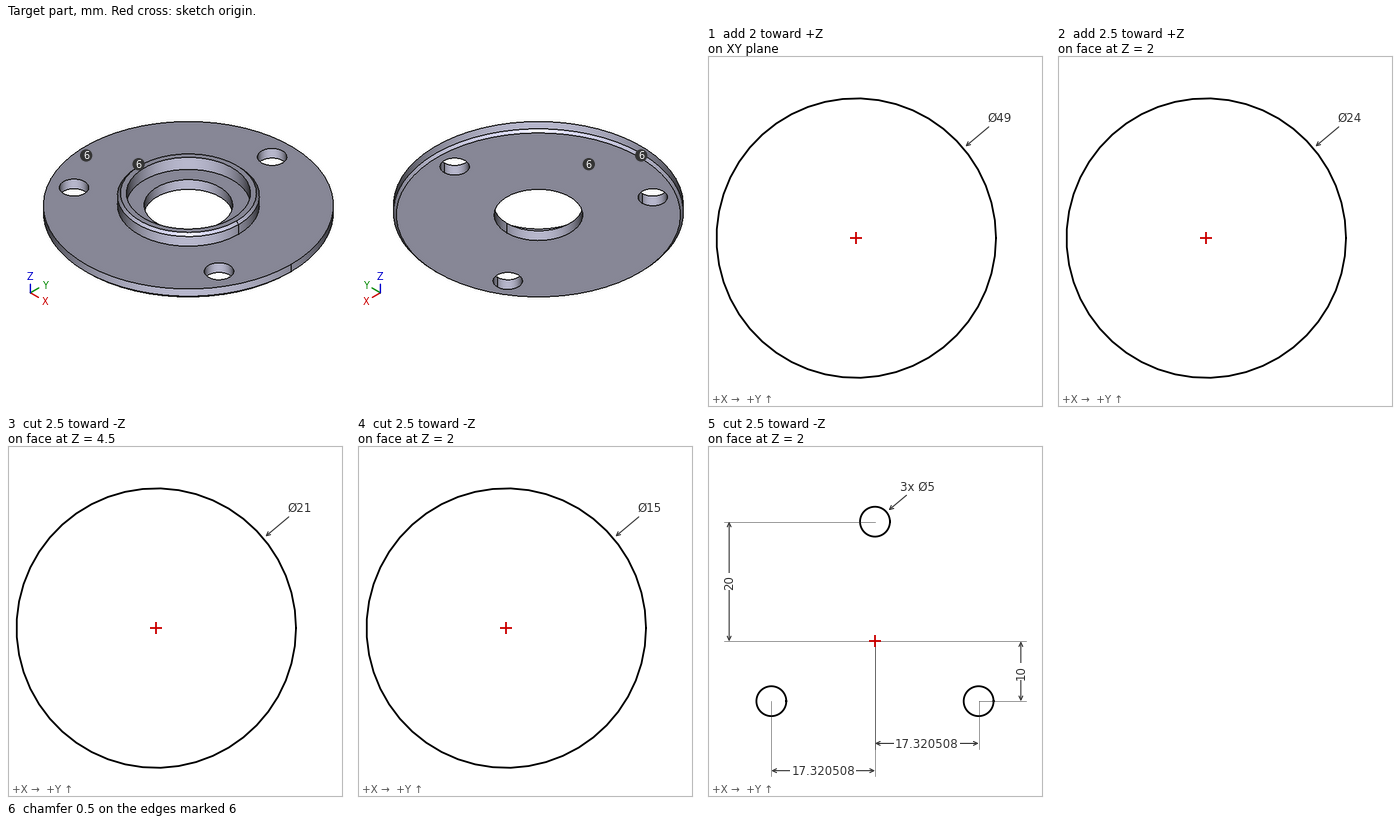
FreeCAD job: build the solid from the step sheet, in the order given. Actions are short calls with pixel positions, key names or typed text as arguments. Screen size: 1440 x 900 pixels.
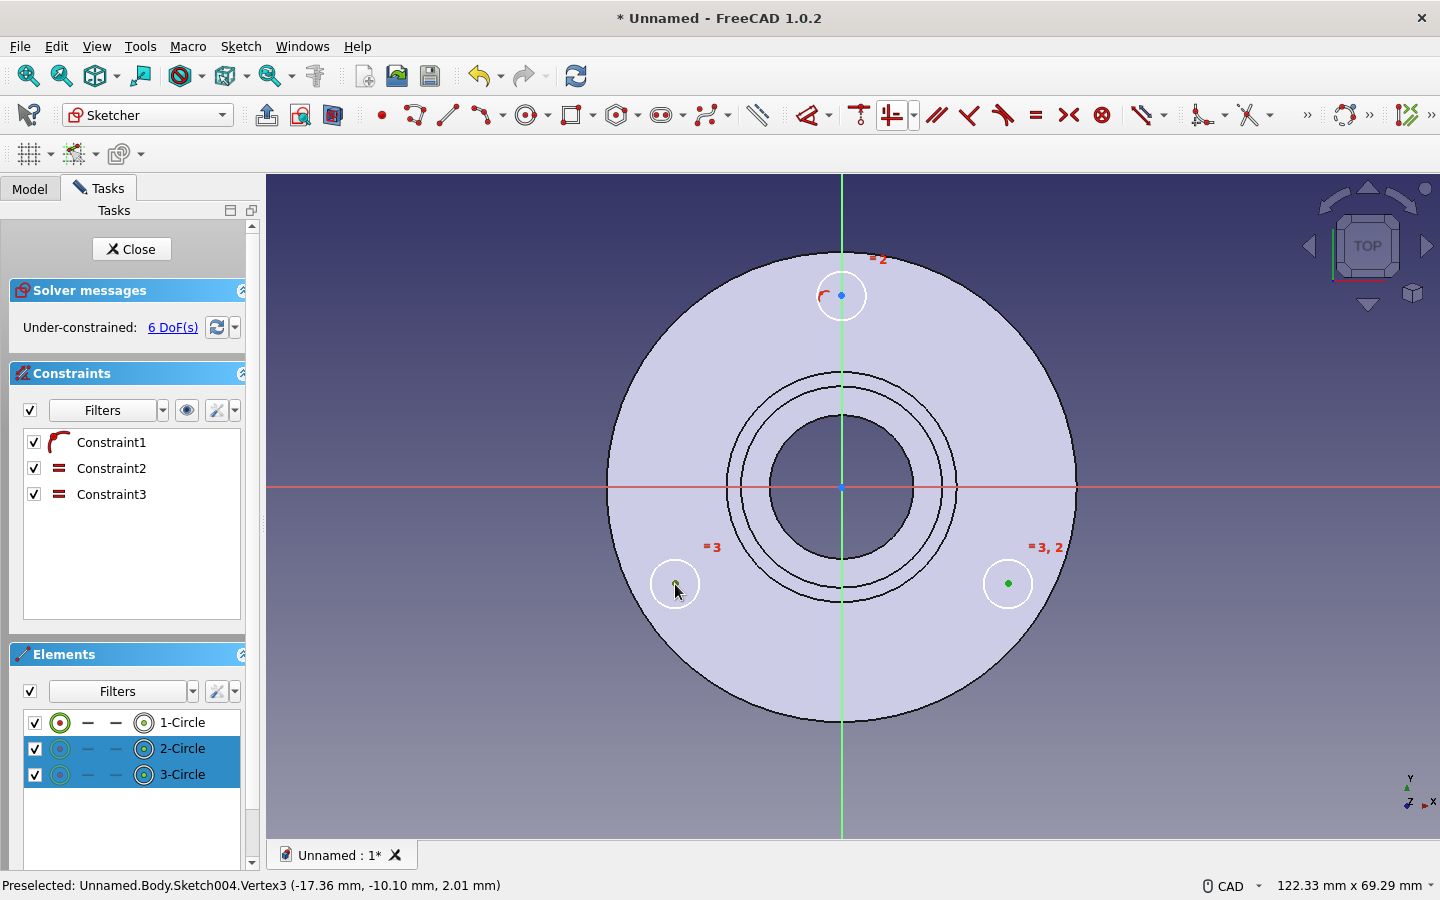
key(h)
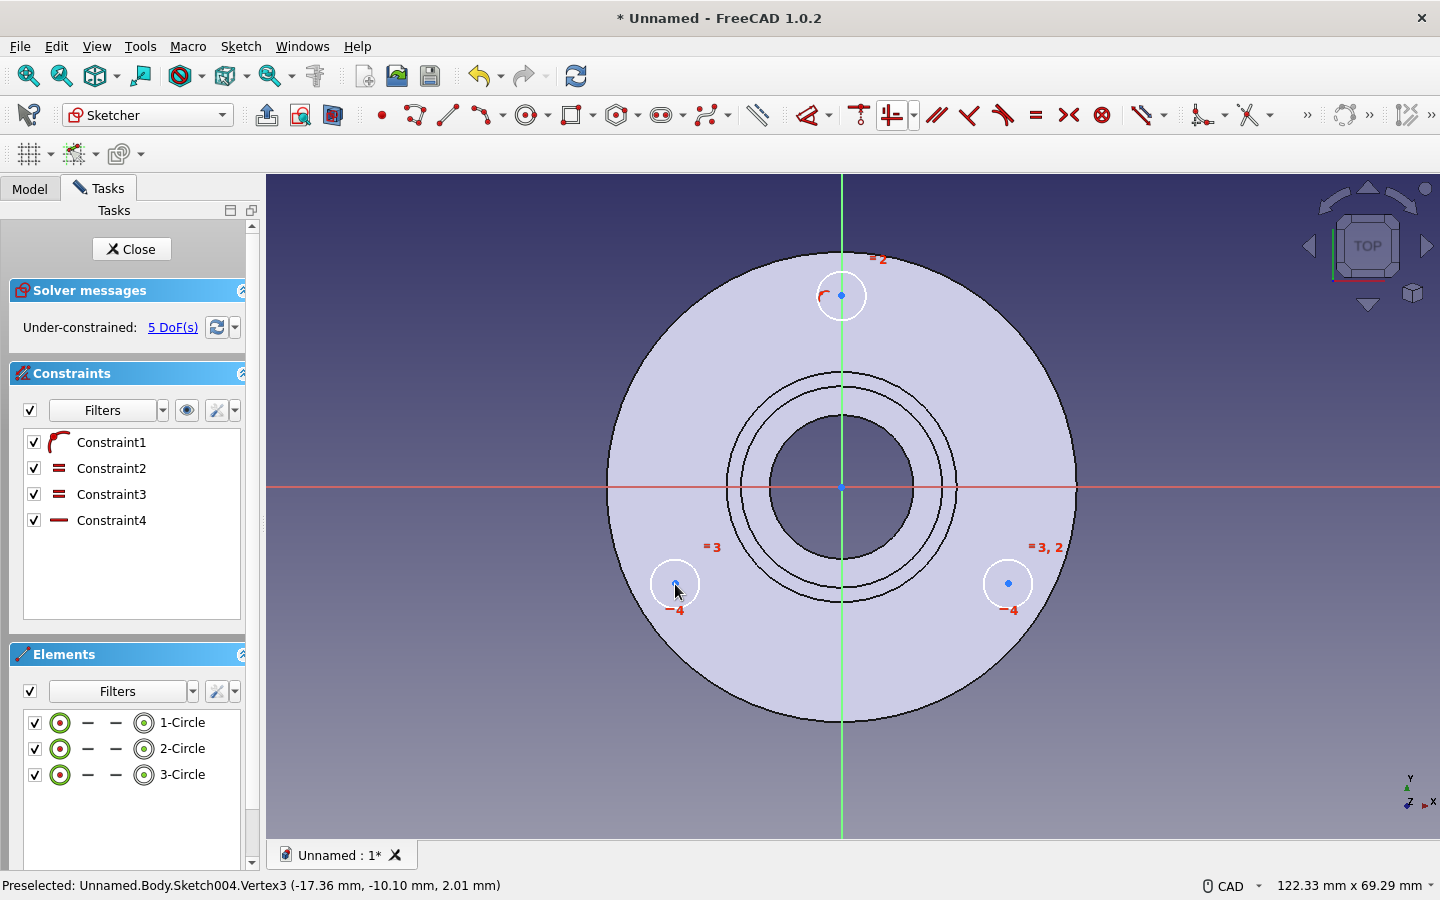
click(859, 279)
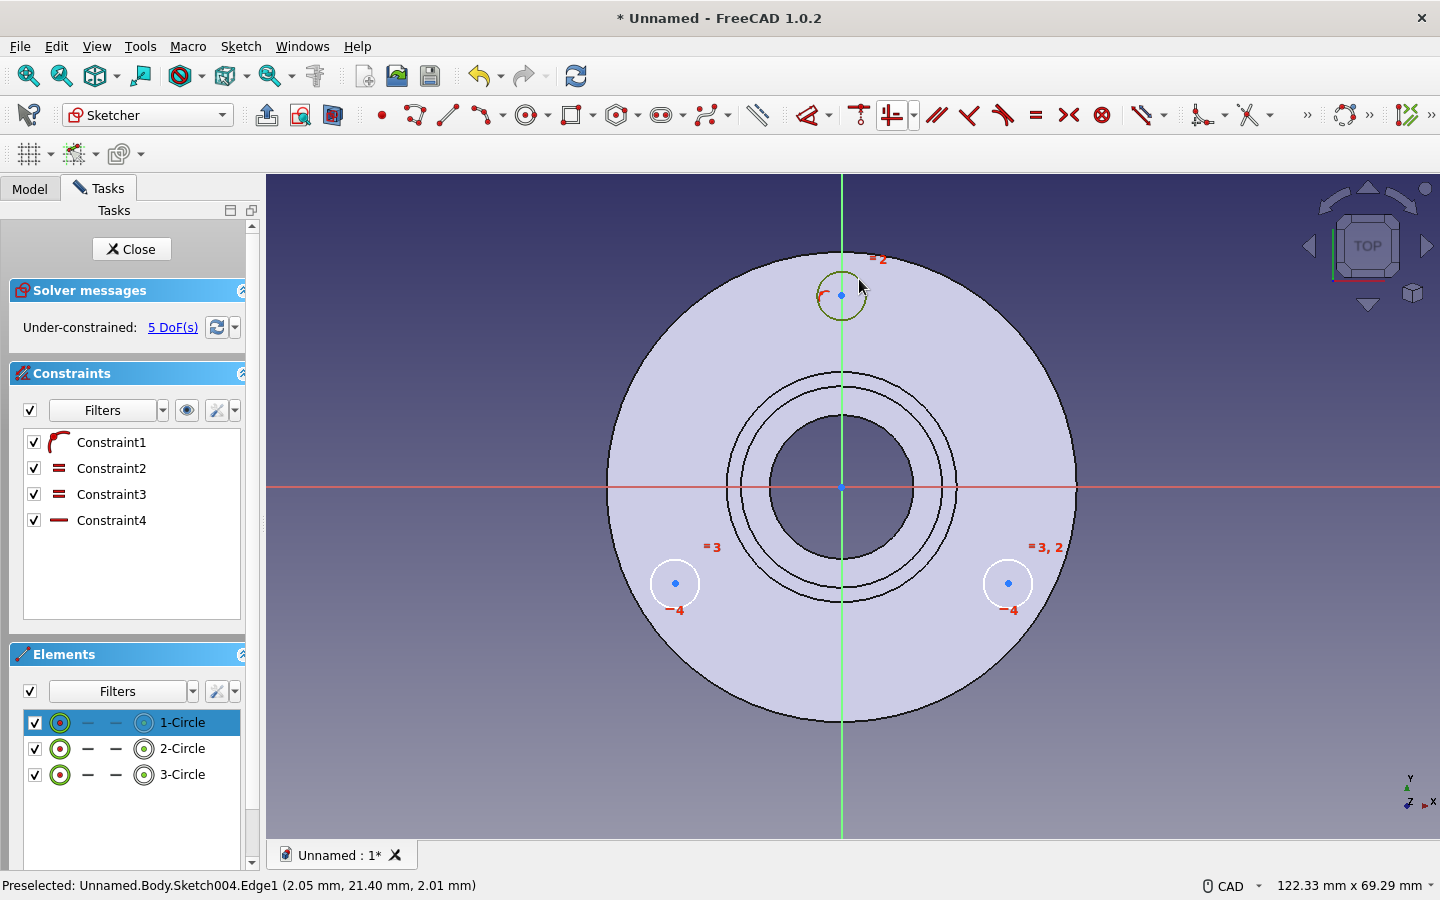
key(k)
key(o)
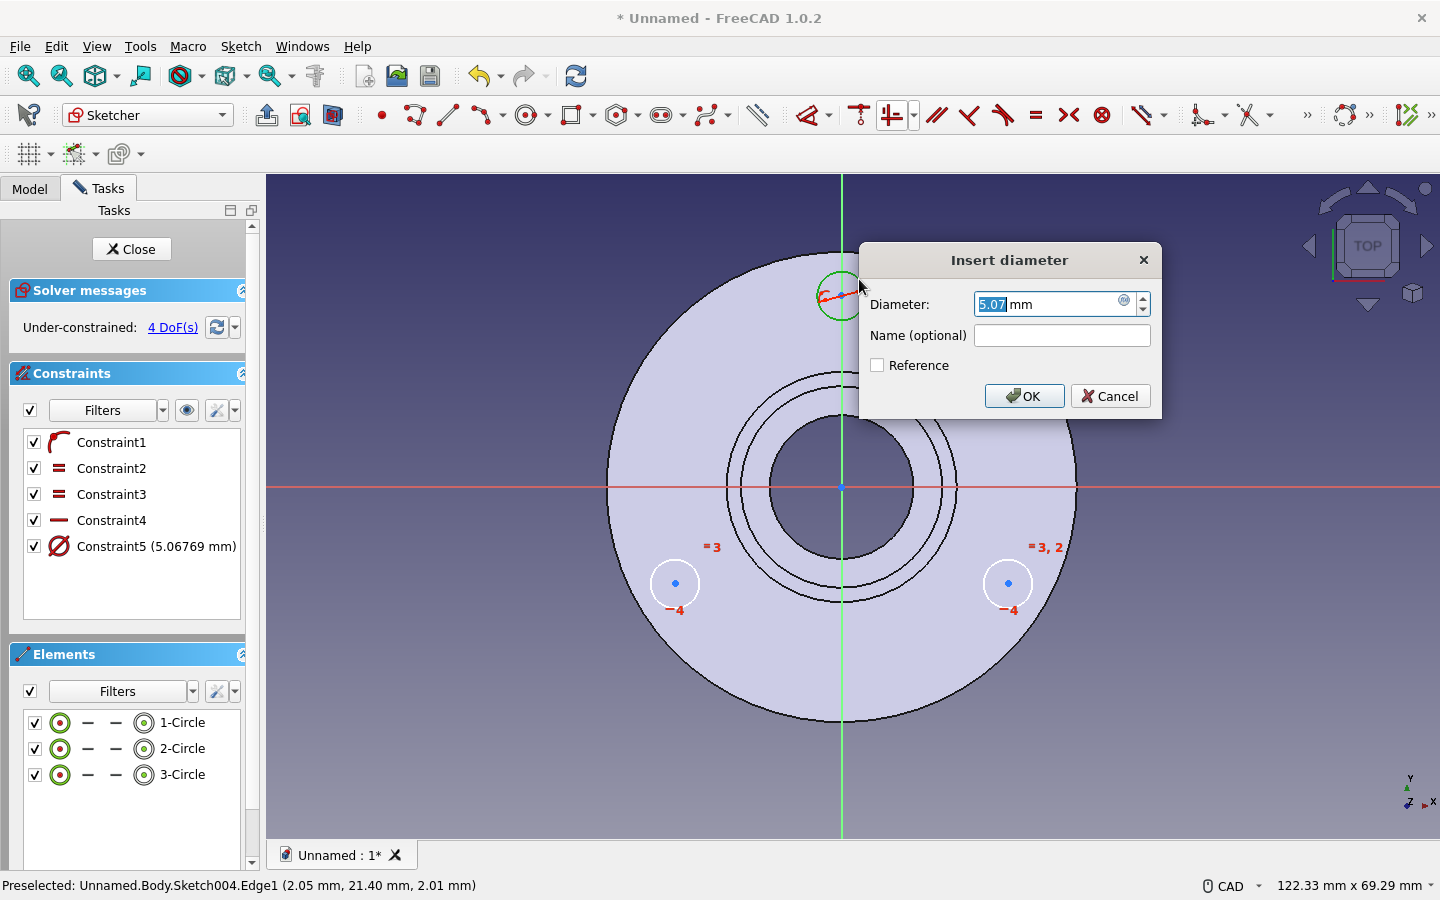
text(5)
key(Return)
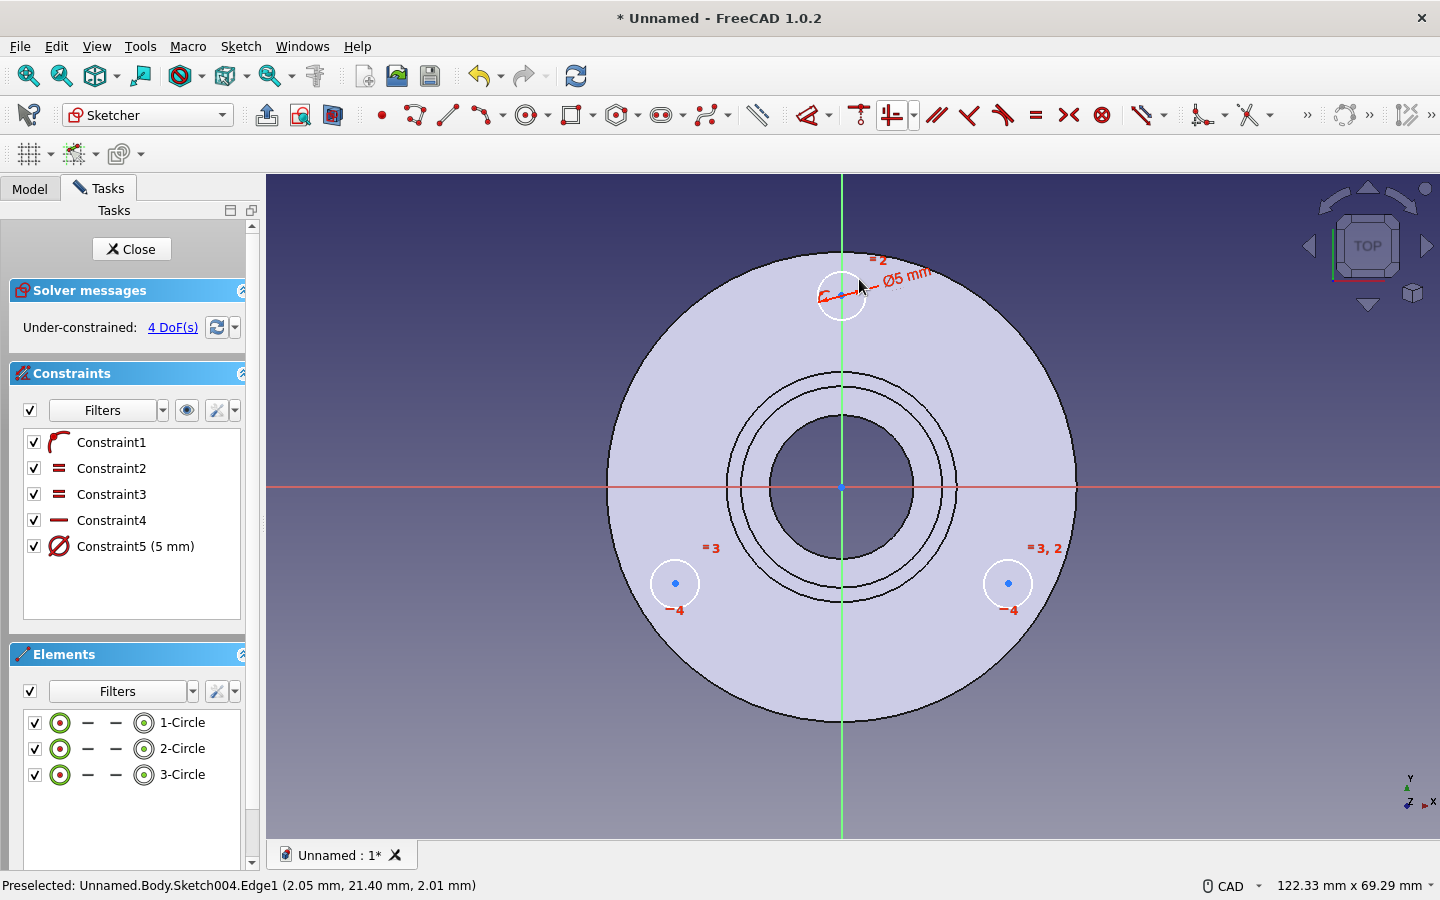
click(842, 296)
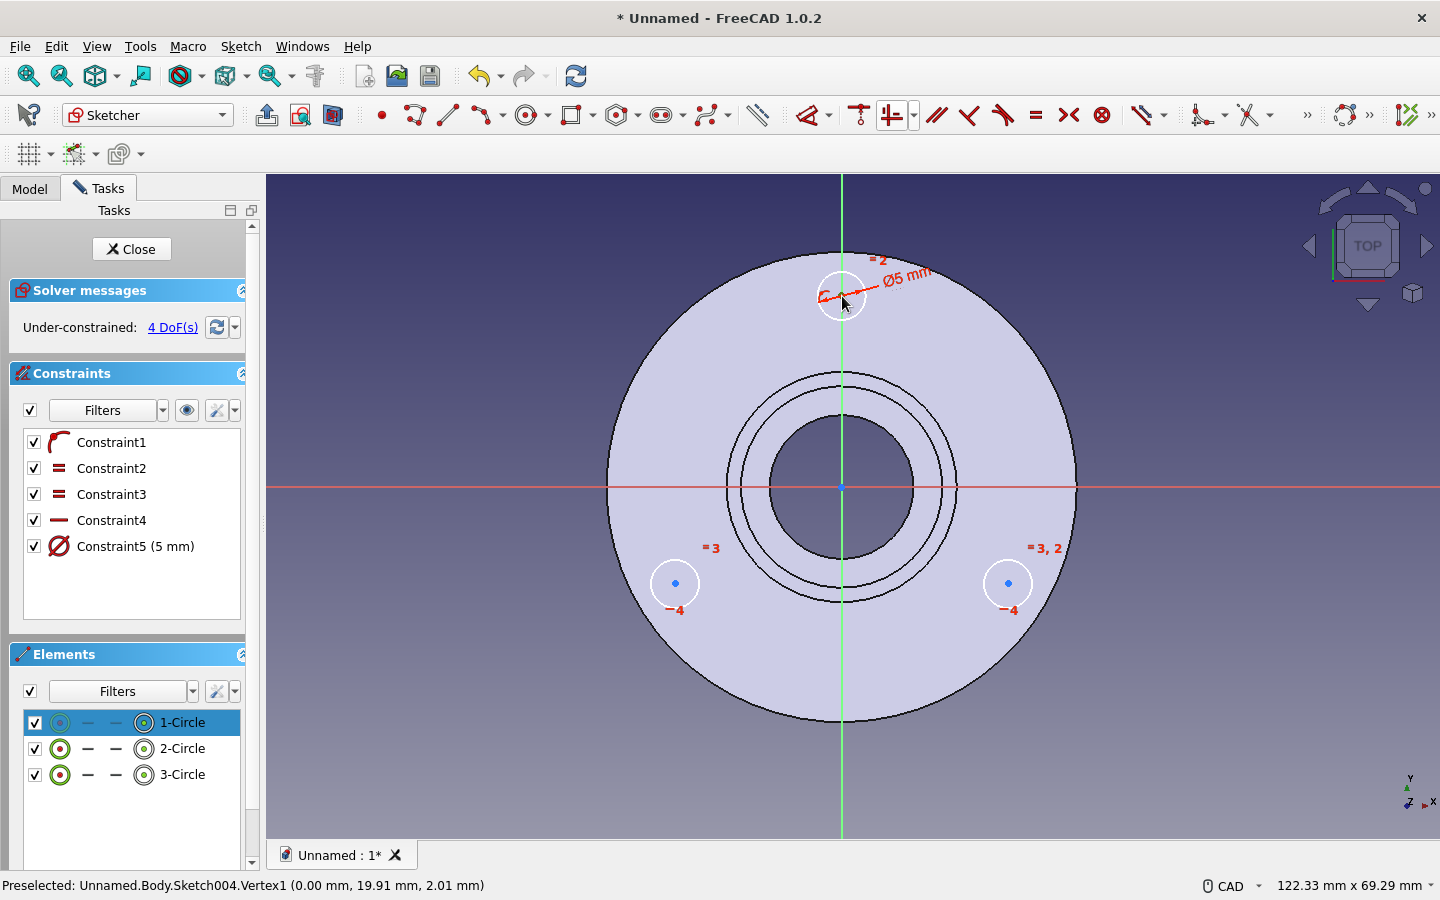
click(828, 116)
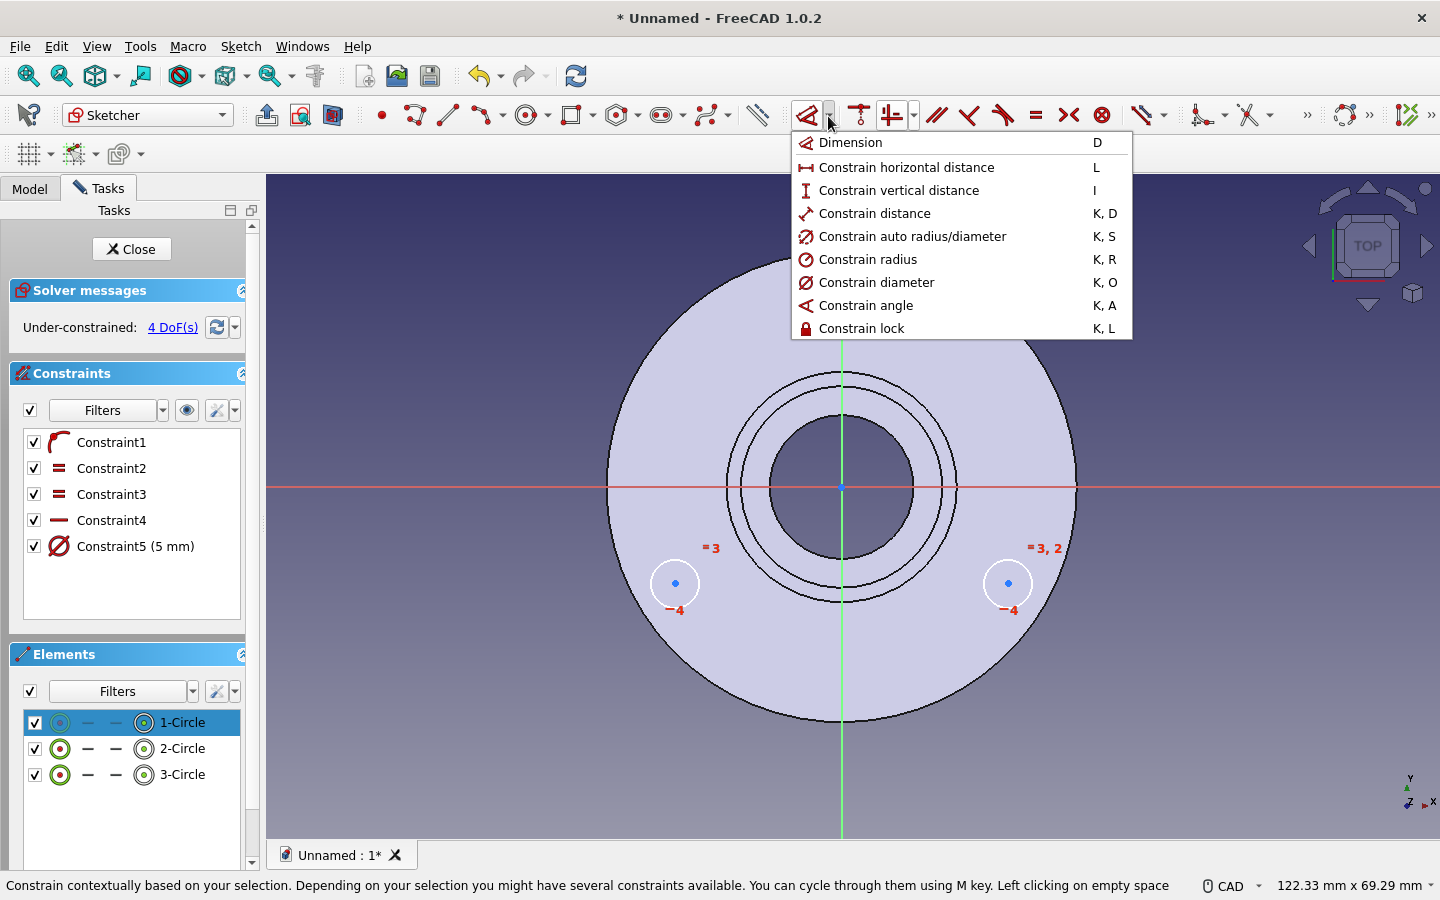
click(962, 190)